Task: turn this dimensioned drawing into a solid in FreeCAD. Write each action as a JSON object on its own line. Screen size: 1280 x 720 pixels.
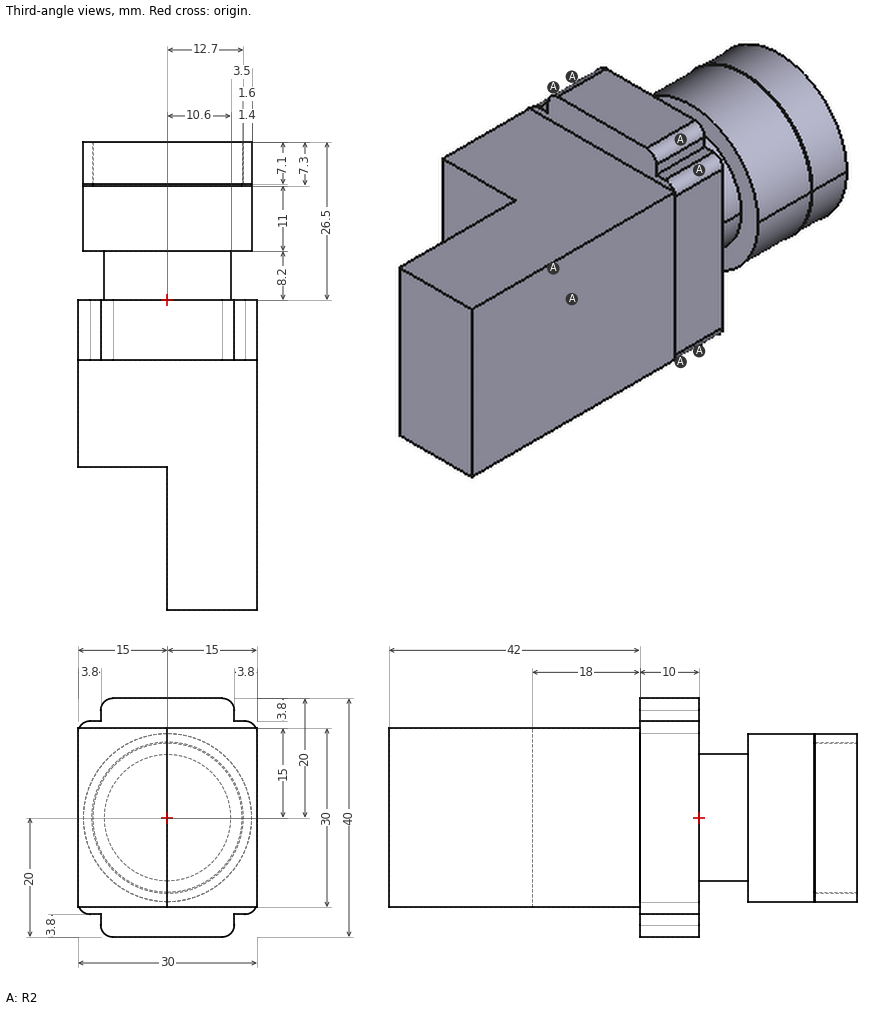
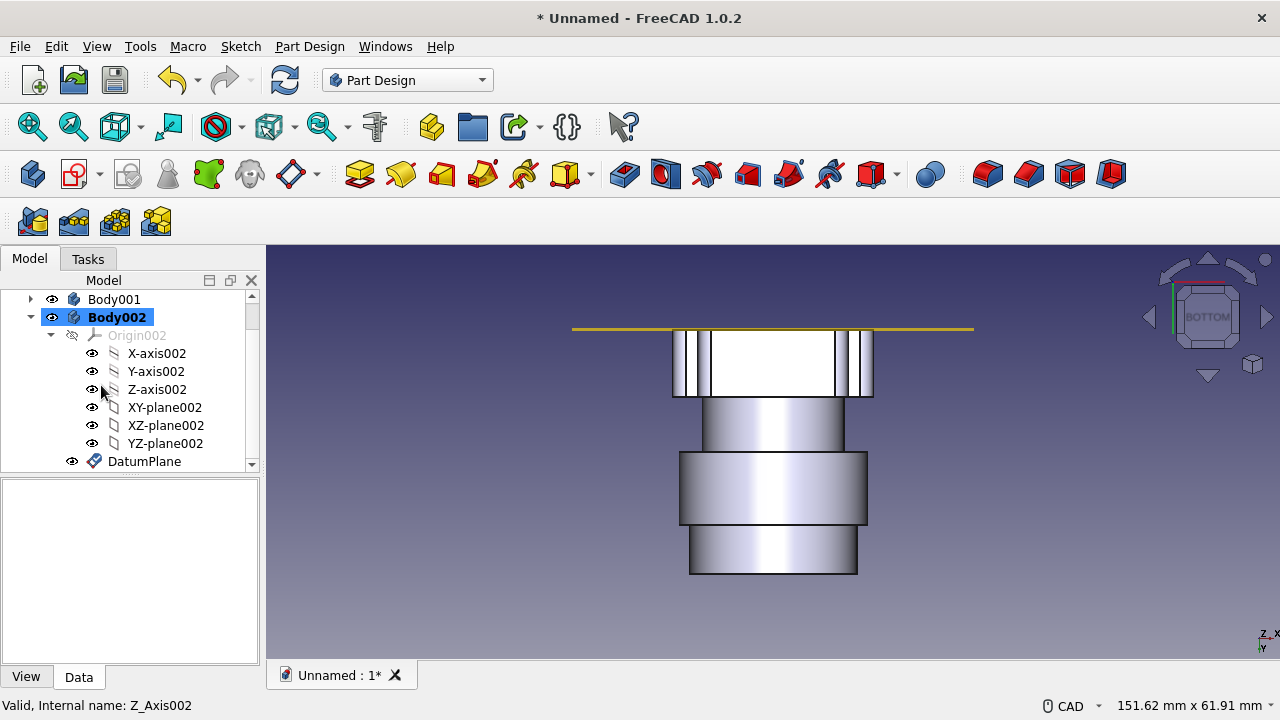
{"action": "left_click", "coordinate": [117, 461]}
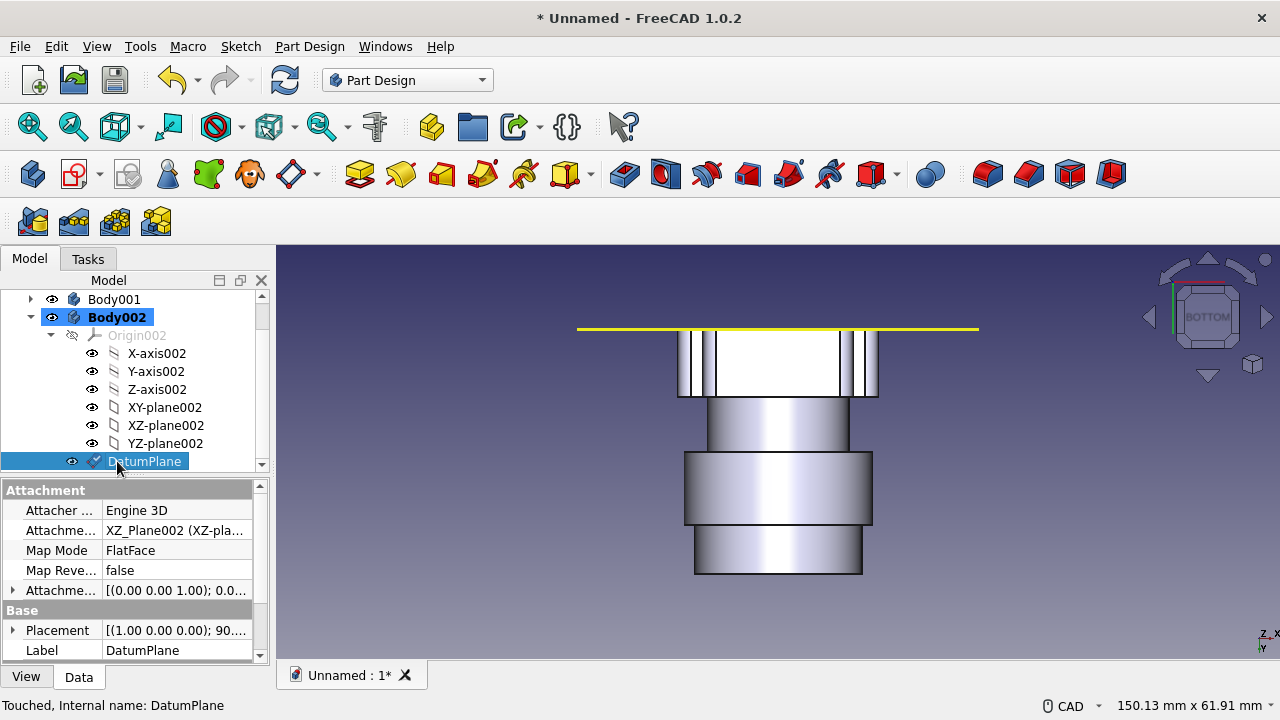
{"action": "left_click", "coordinate": [74, 174]}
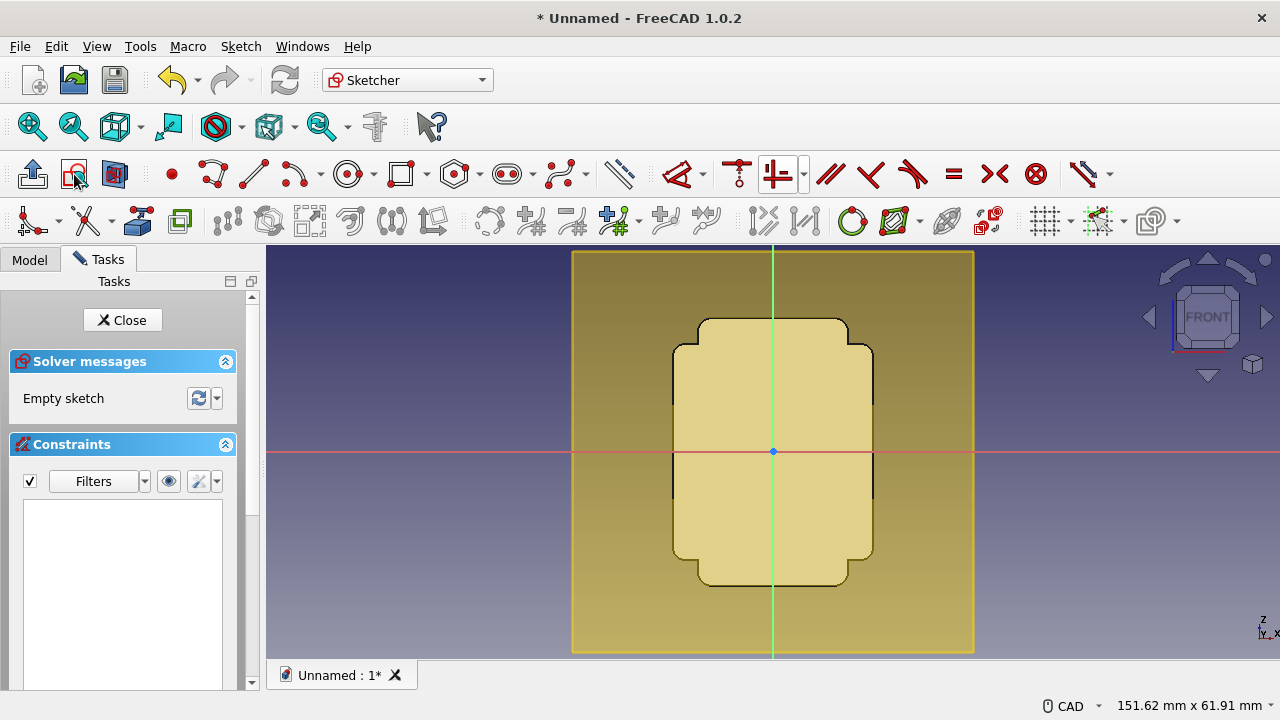
{"action": "left_click", "coordinate": [400, 174]}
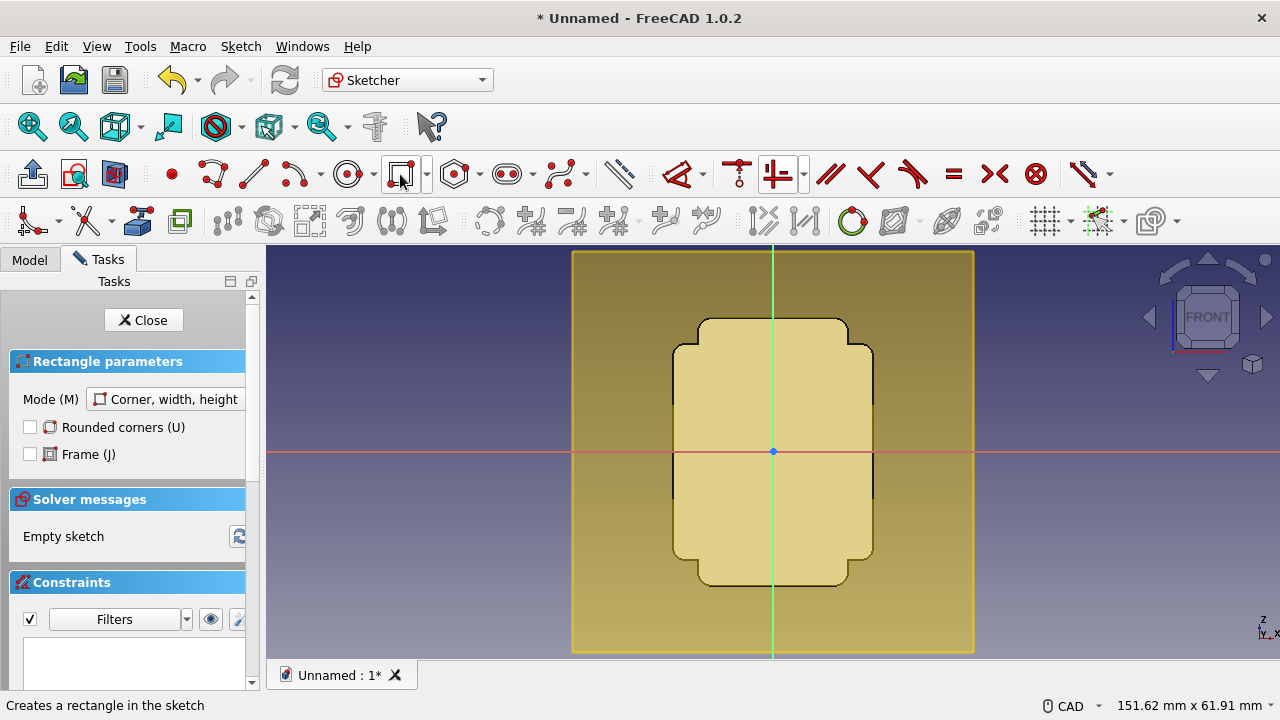
{"action": "left_click", "coordinate": [773, 352]}
{"action": "mouse_move", "coordinate": [873, 552]}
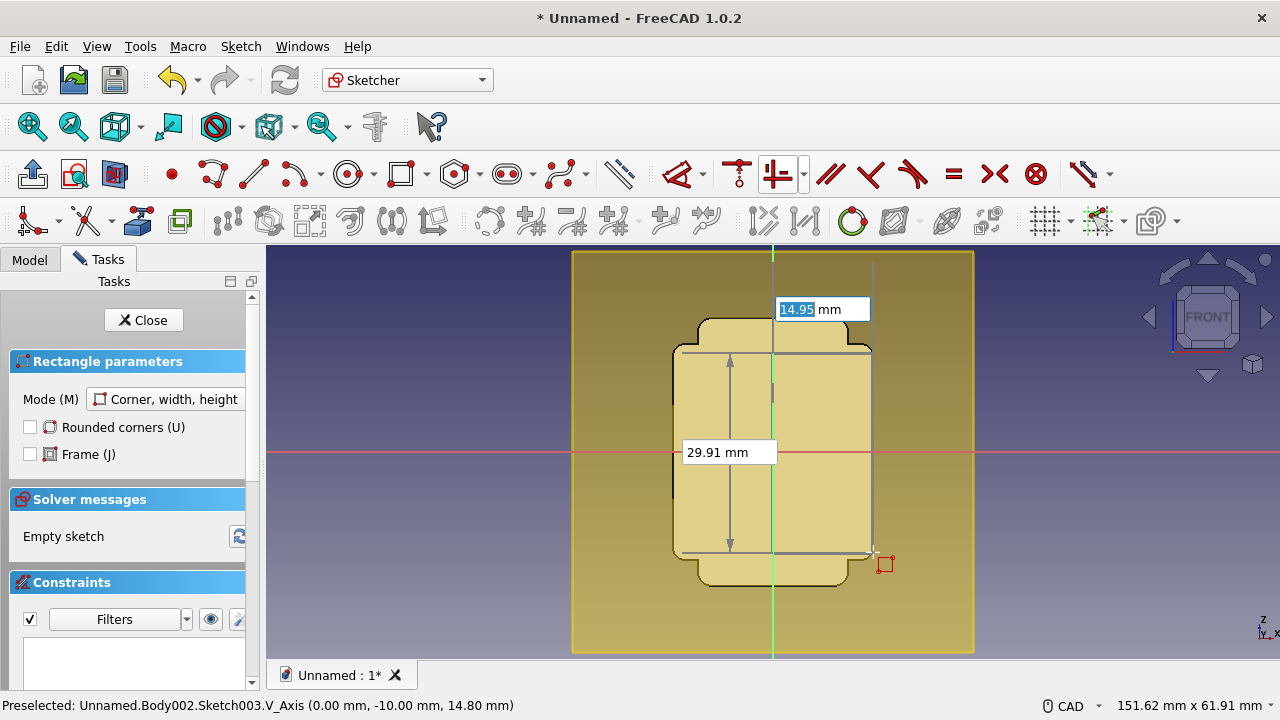
{"action": "type", "text": "15"}
{"action": "key", "text": "Tab"}
{"action": "type", "text": "30"}
{"action": "key", "text": "Return"}
{"action": "key", "text": "Escape"}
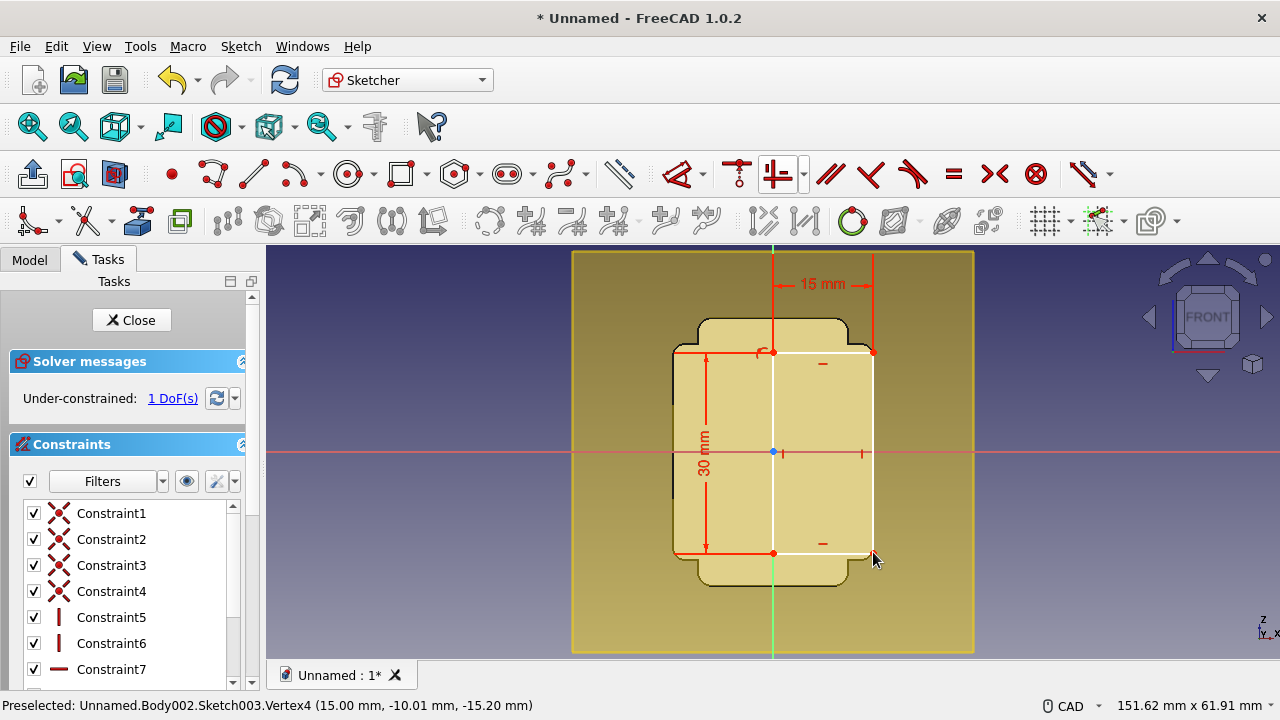
{"action": "key", "text": "d"}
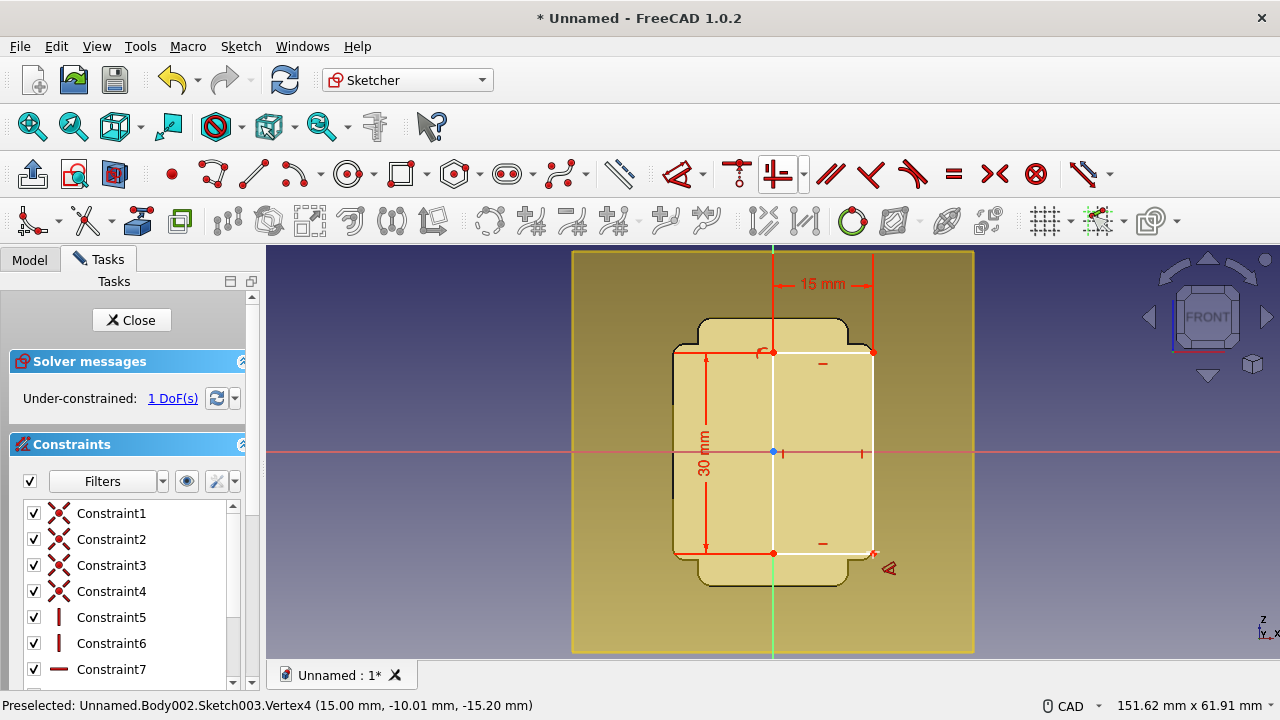
{"action": "left_click", "coordinate": [773, 353]}
{"action": "left_click", "coordinate": [739, 403]}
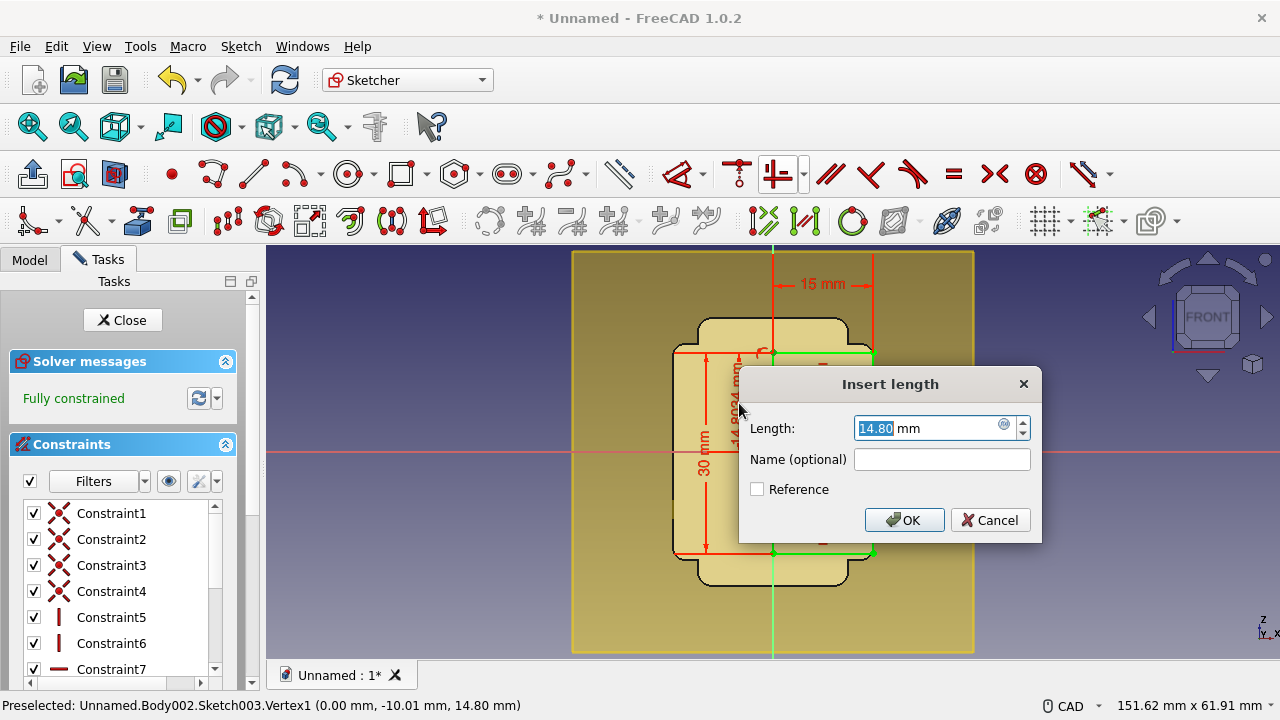
{"action": "type", "text": "15"}
{"action": "key", "text": "Return"}
{"action": "key", "text": "Escape"}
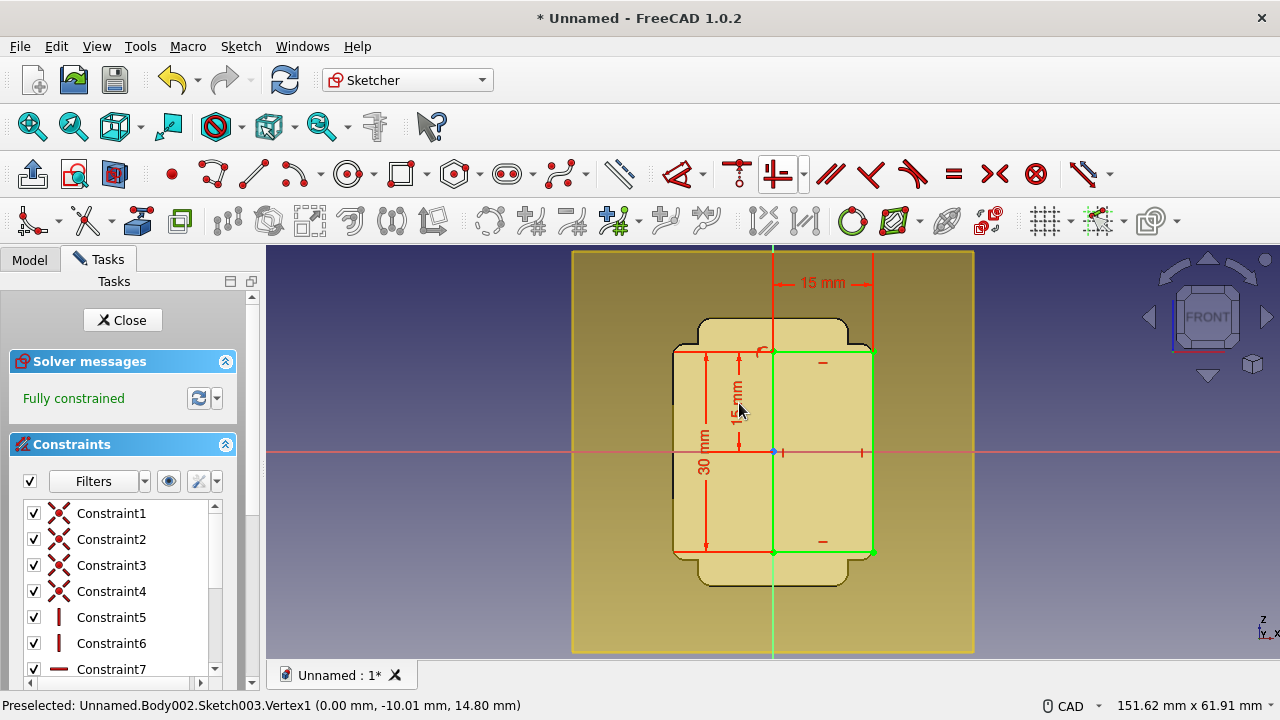
{"action": "left_click", "coordinate": [123, 320]}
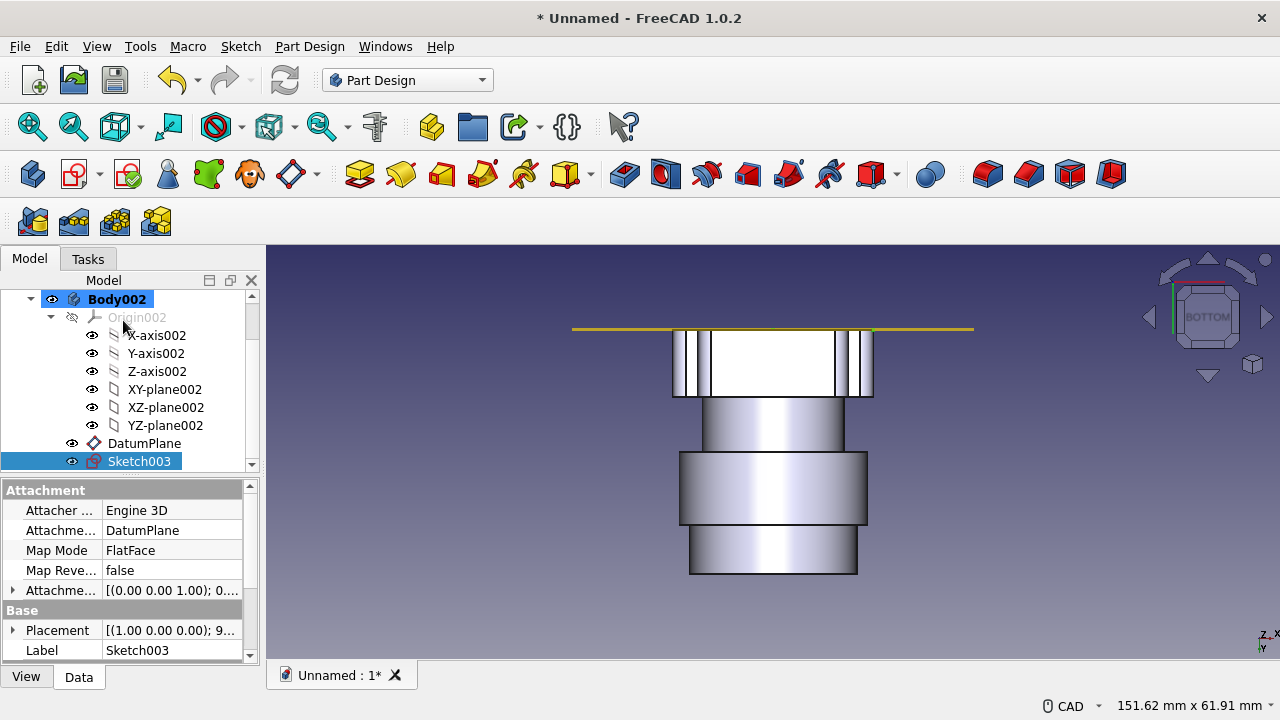
{"action": "left_click", "coordinate": [360, 174]}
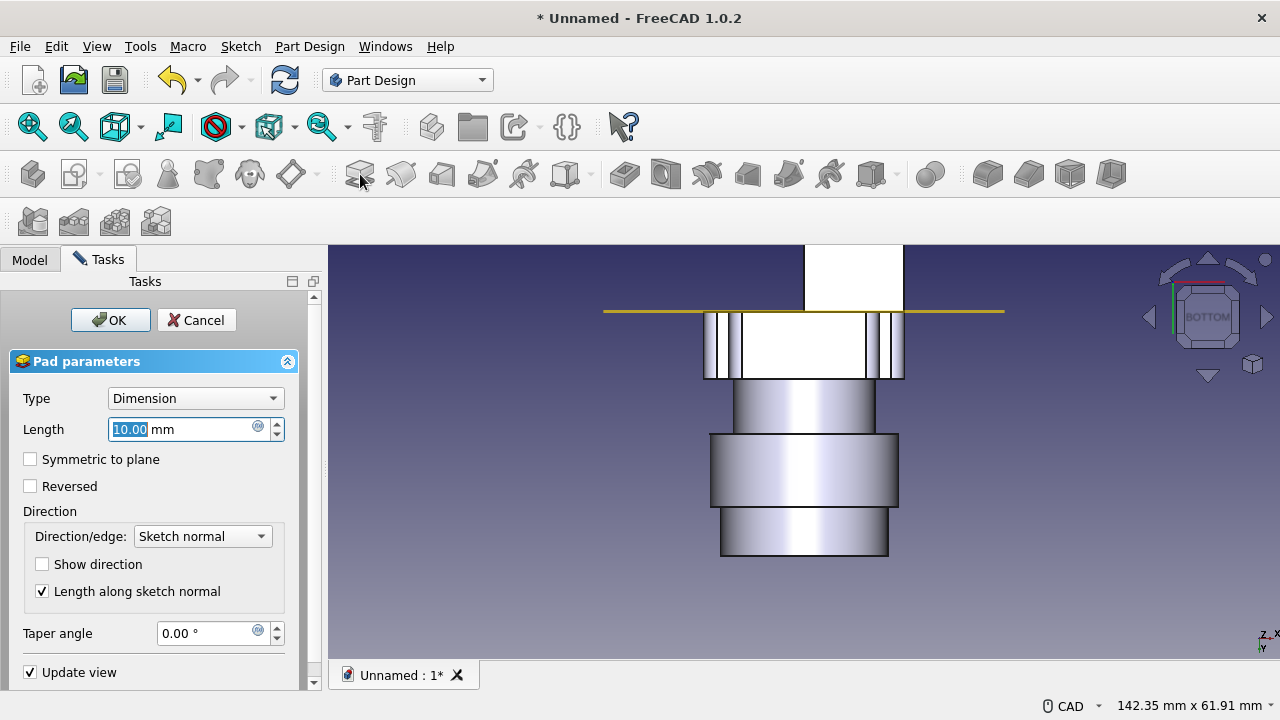
{"action": "type", "text": "42"}
{"action": "key", "text": "Tab"}